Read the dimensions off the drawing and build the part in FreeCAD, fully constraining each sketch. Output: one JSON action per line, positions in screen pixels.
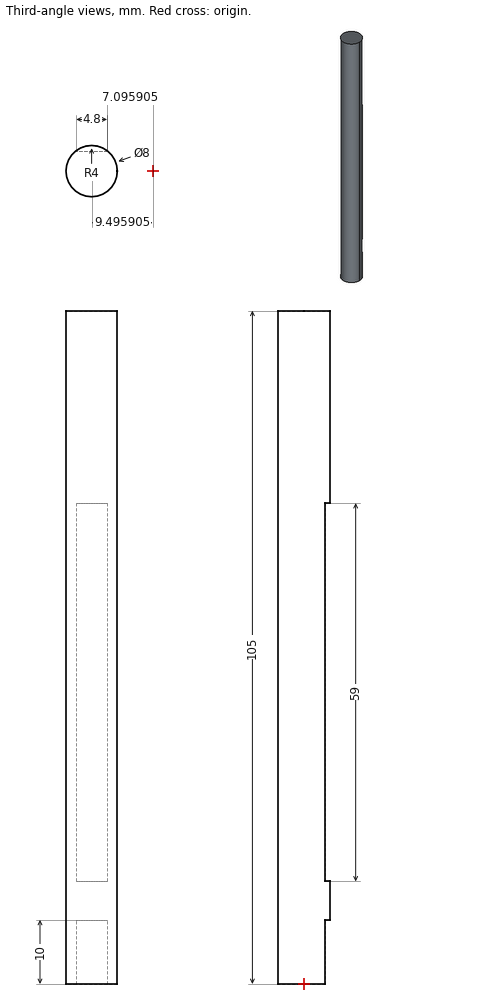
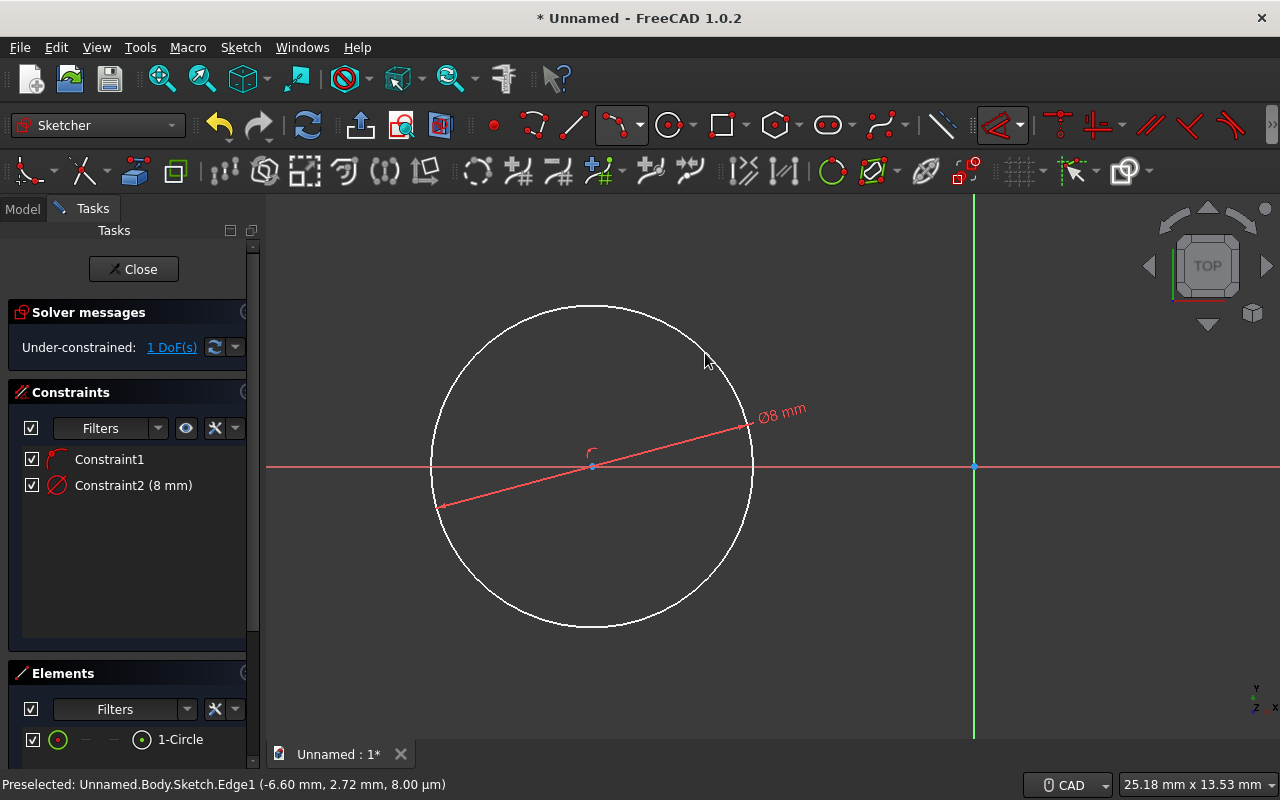
{"action": "left_click", "coordinate": [592, 466]}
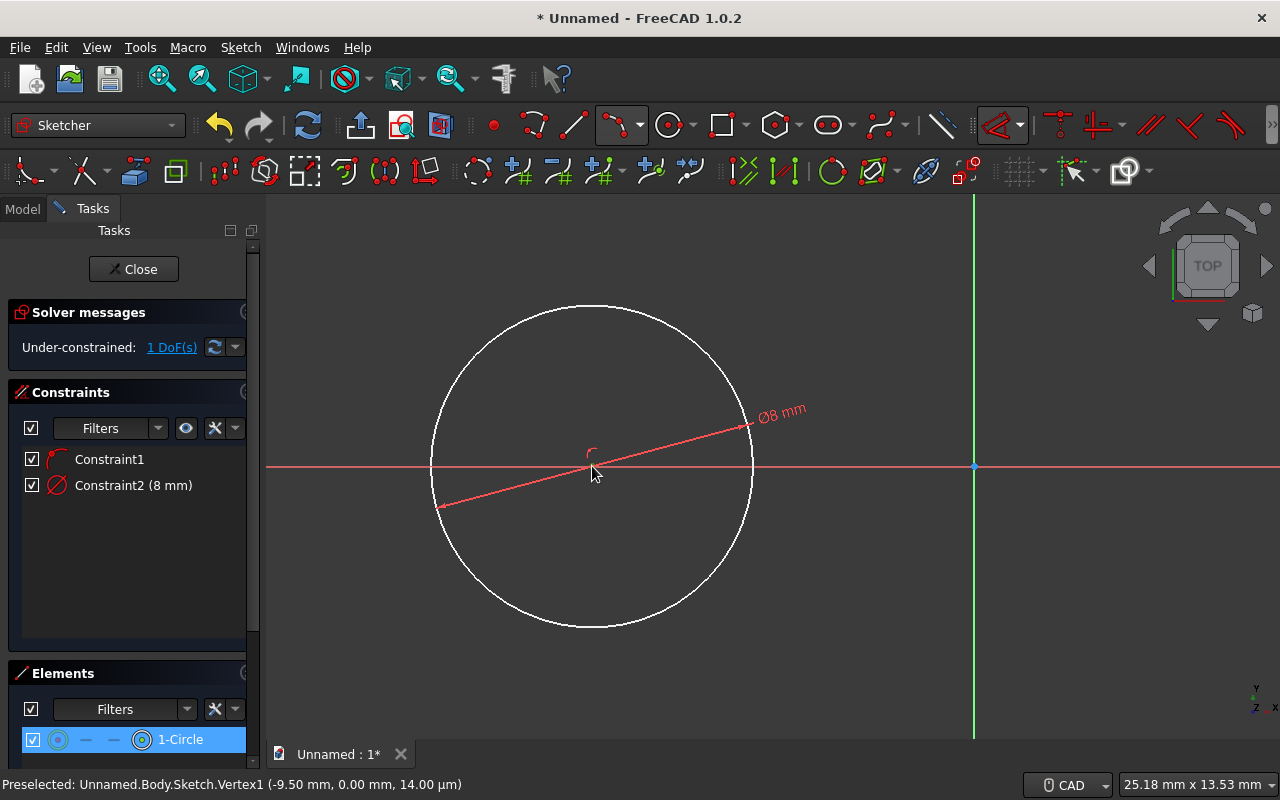
{"action": "key", "text": "l"}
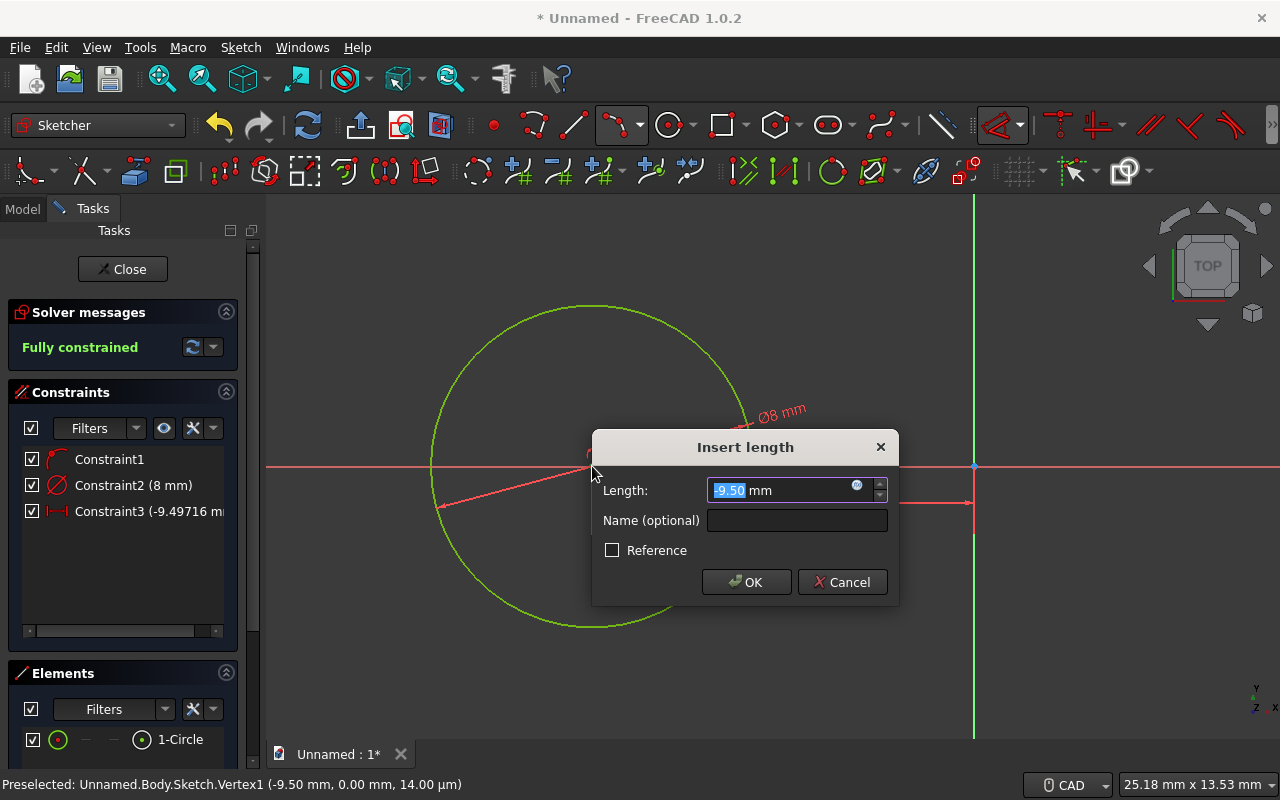
{"action": "type", "text": "-9.495905"}
{"action": "key", "text": "Return"}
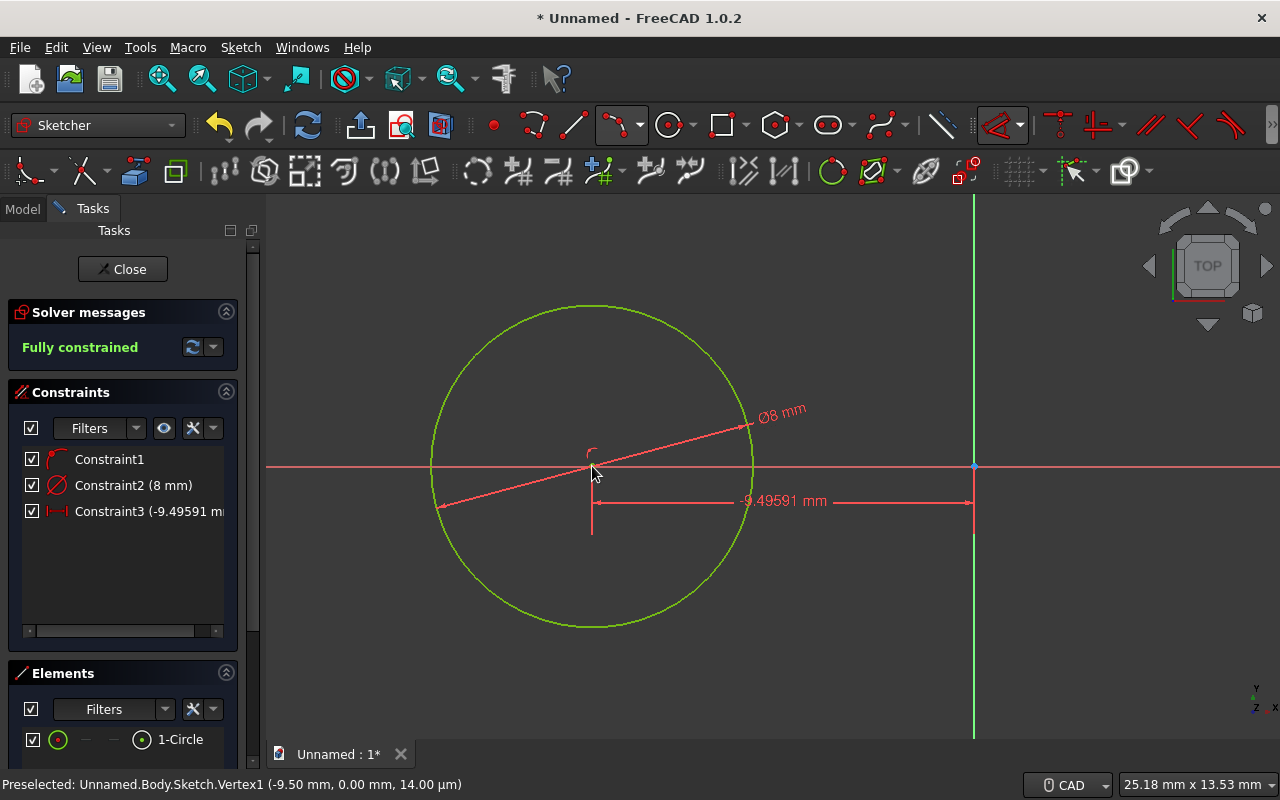
{"action": "left_click", "coordinate": [123, 269]}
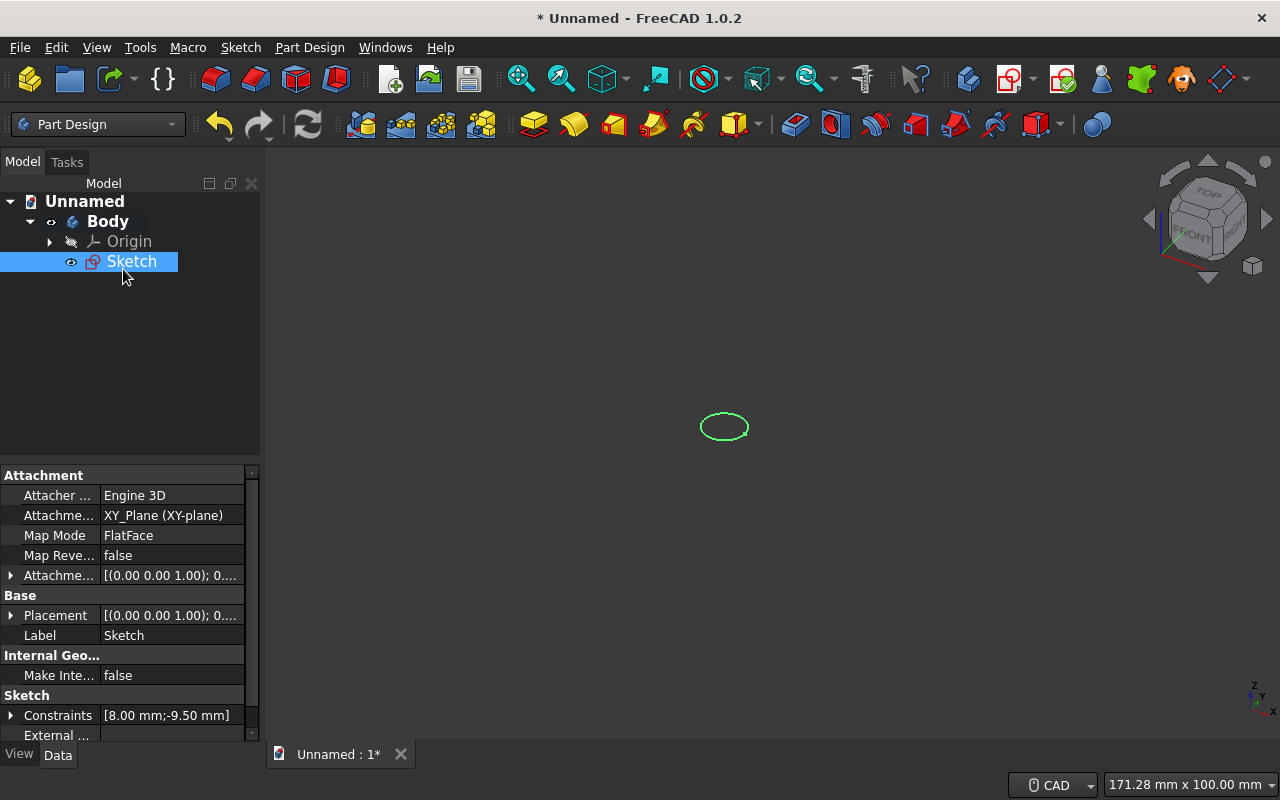
{"action": "left_click", "coordinate": [534, 124]}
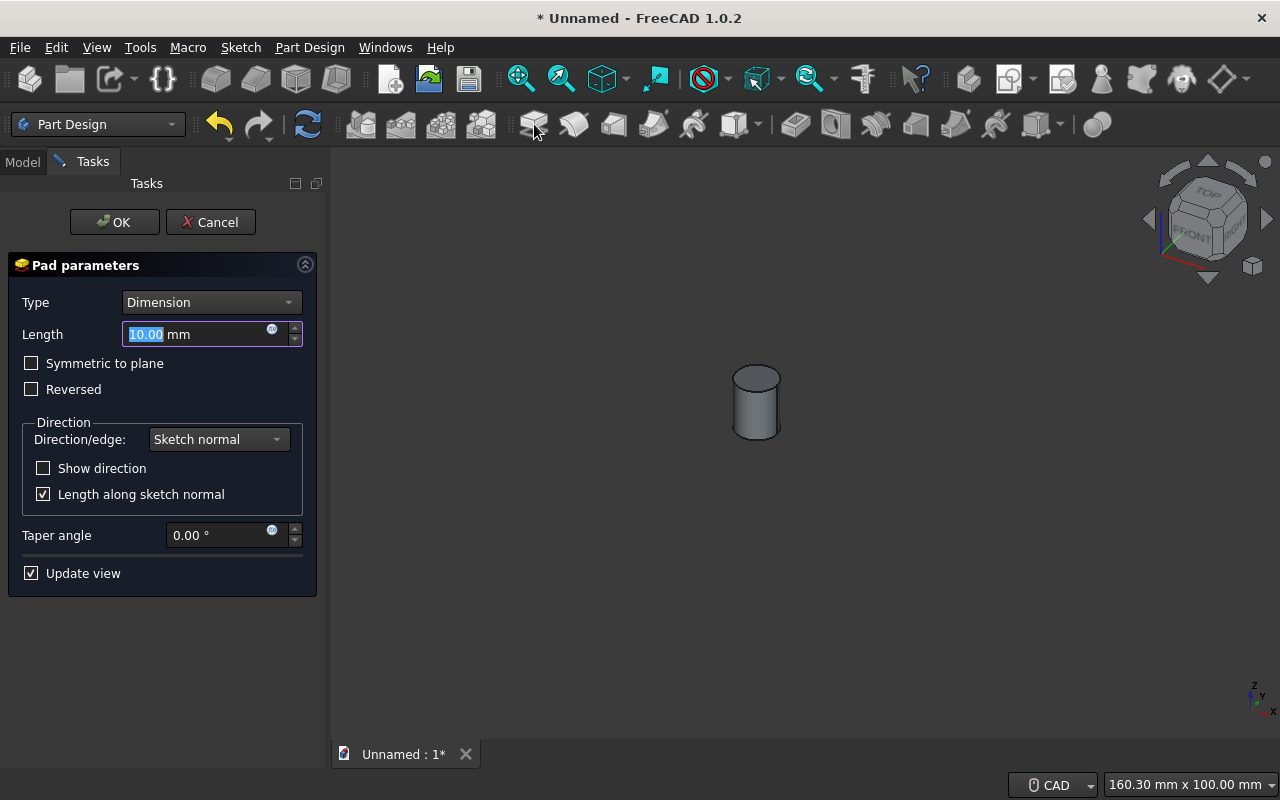
{"action": "type", "text": "105"}
{"action": "key", "text": "Tab"}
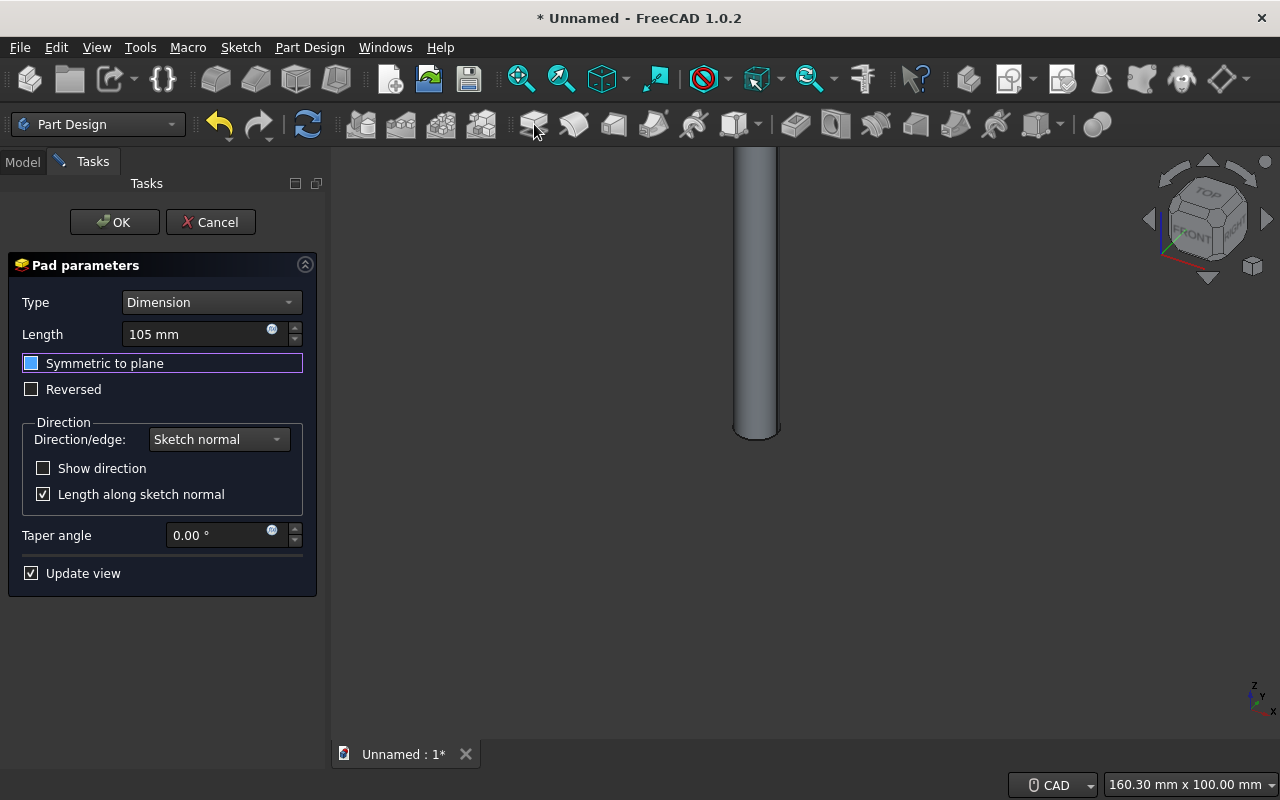
{"action": "left_click", "coordinate": [115, 222]}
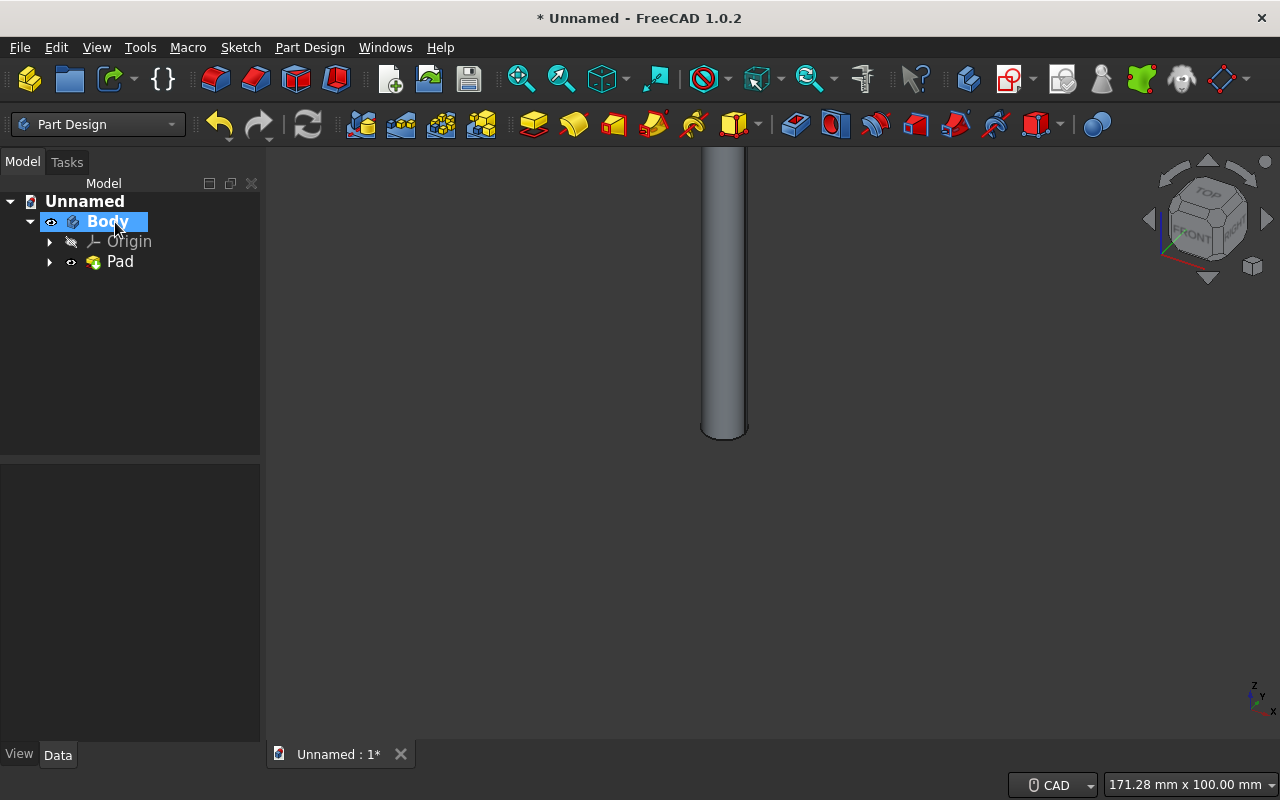
{"action": "key", "text": "v f"}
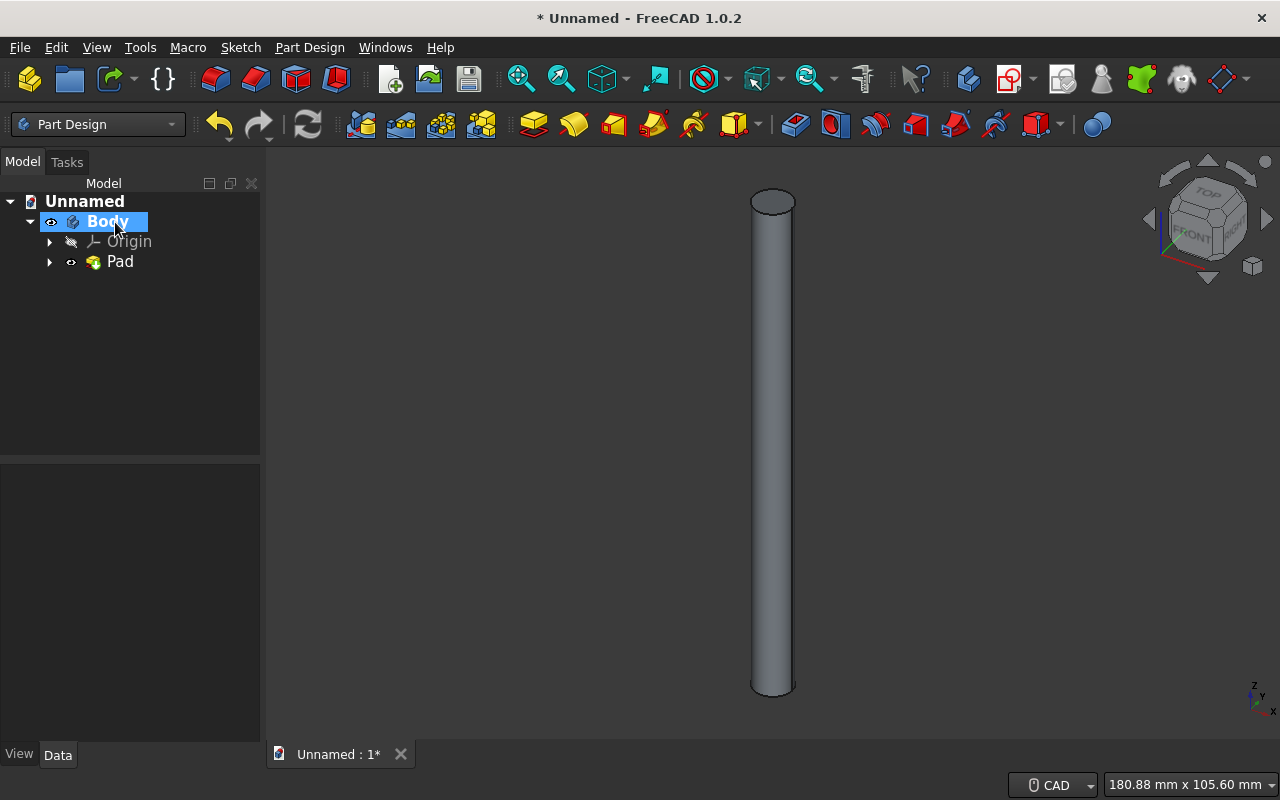
{"action": "left_click", "coordinate": [1010, 80]}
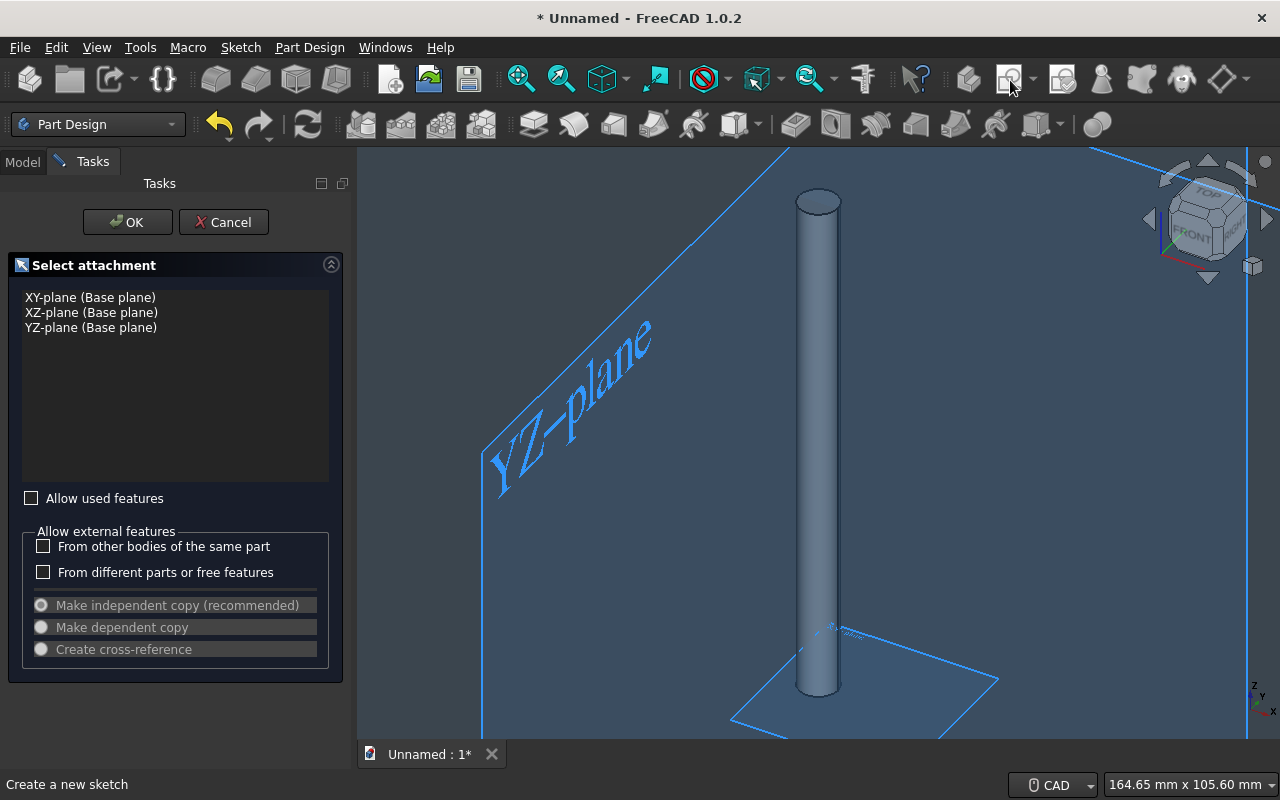
{"action": "left_click", "coordinate": [82, 298]}